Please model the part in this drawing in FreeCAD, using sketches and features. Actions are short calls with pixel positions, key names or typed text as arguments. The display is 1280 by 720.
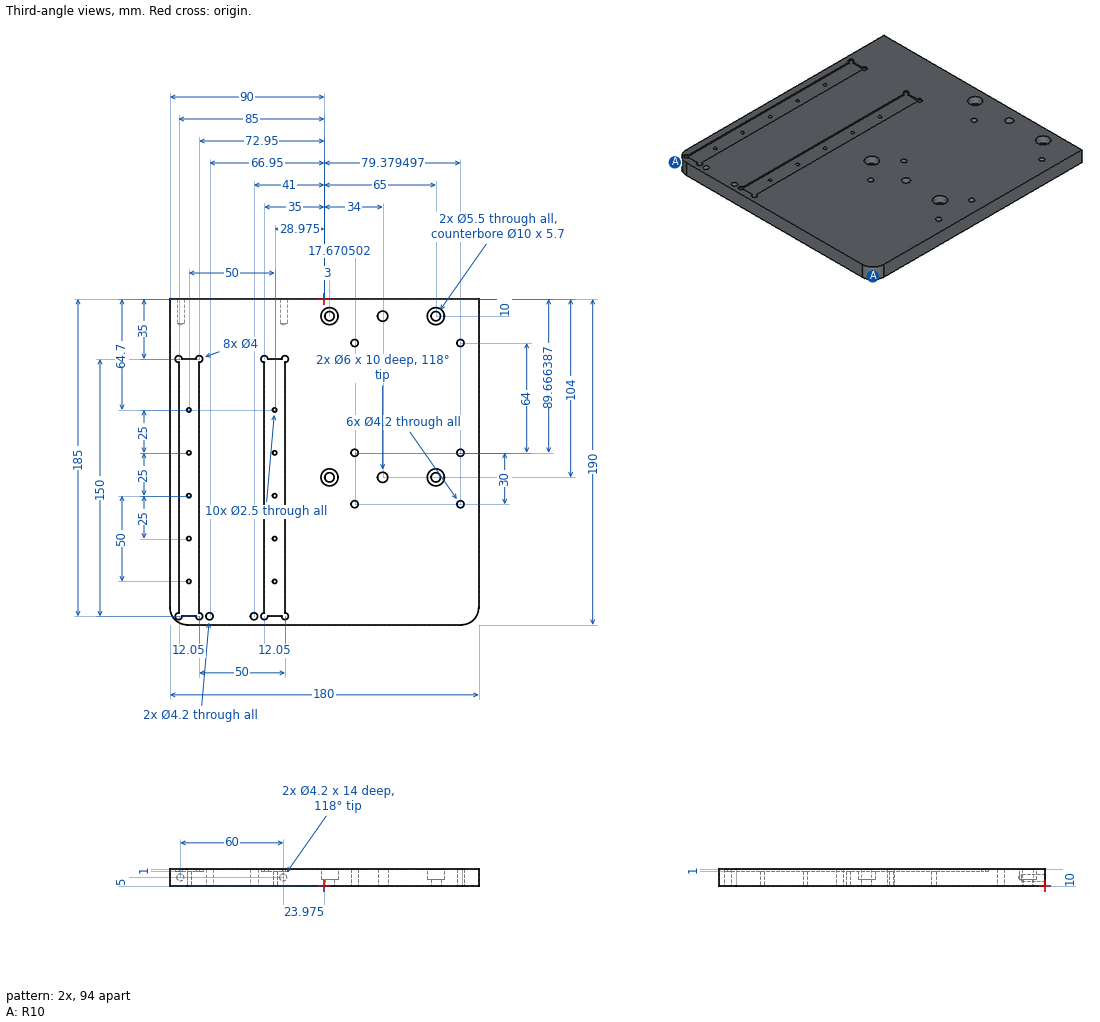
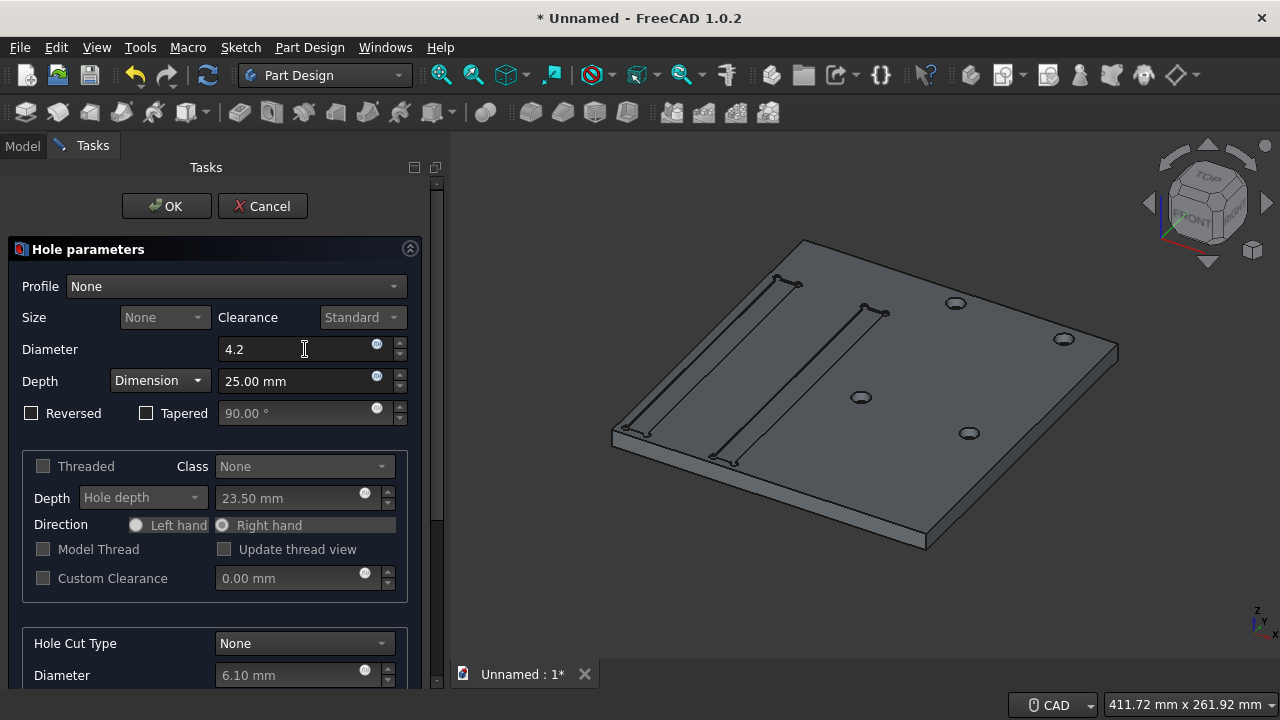
triple_click(305, 381)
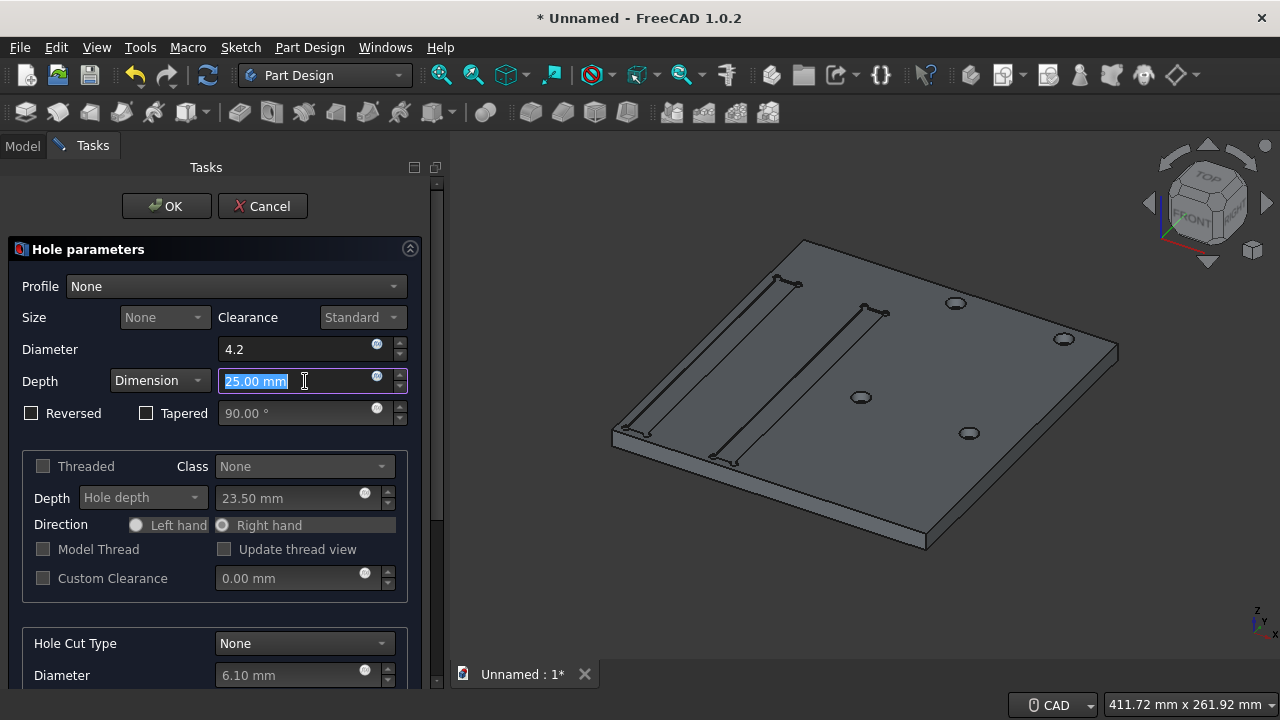
text(14)
key(Tab)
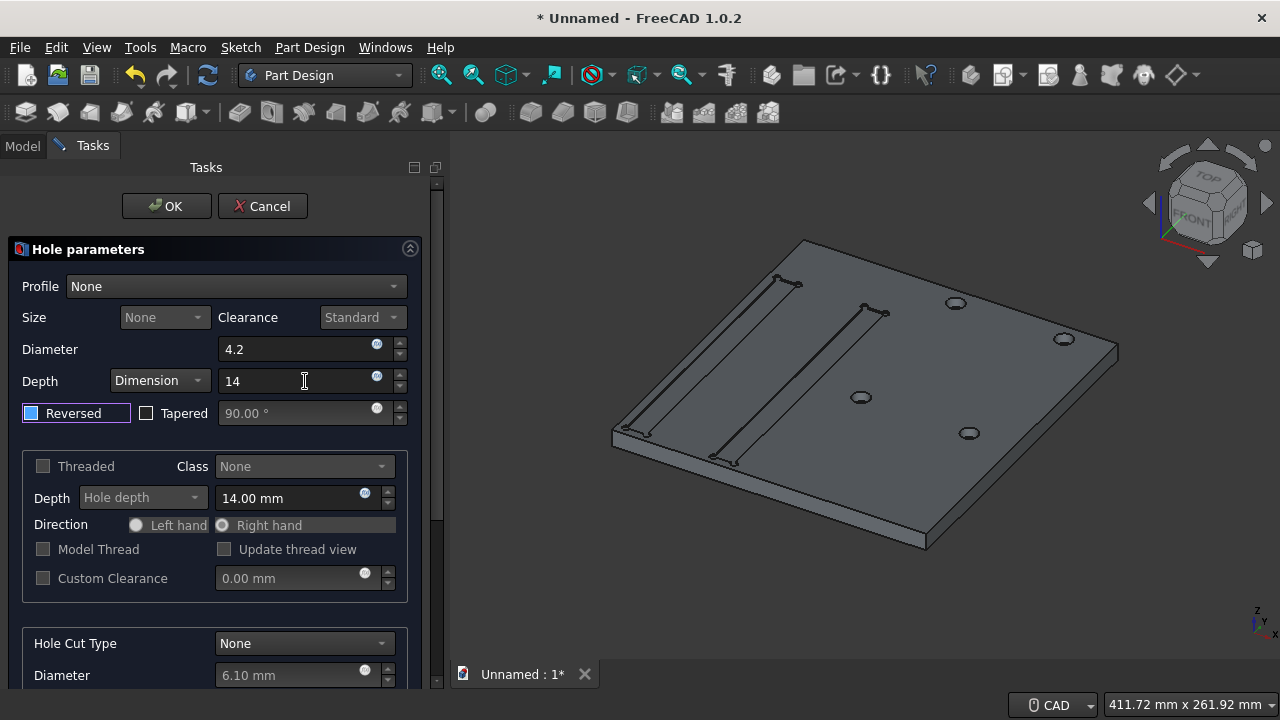
click(30, 413)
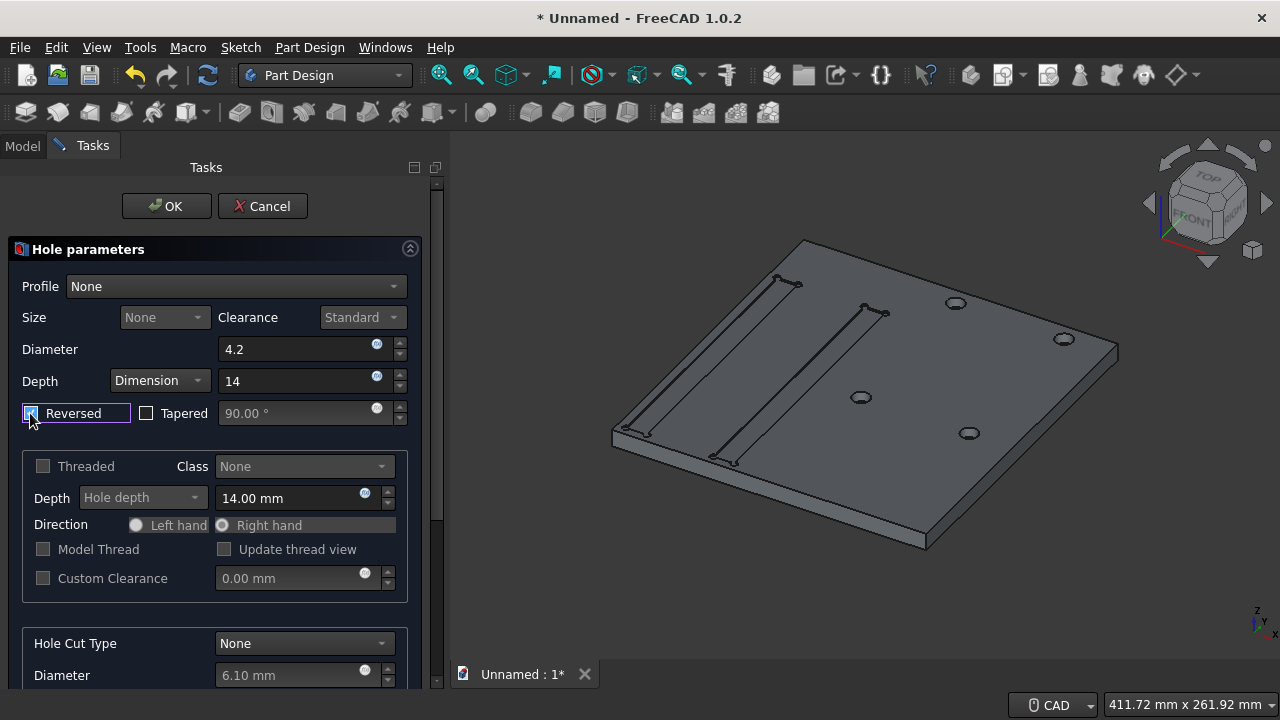
click(167, 206)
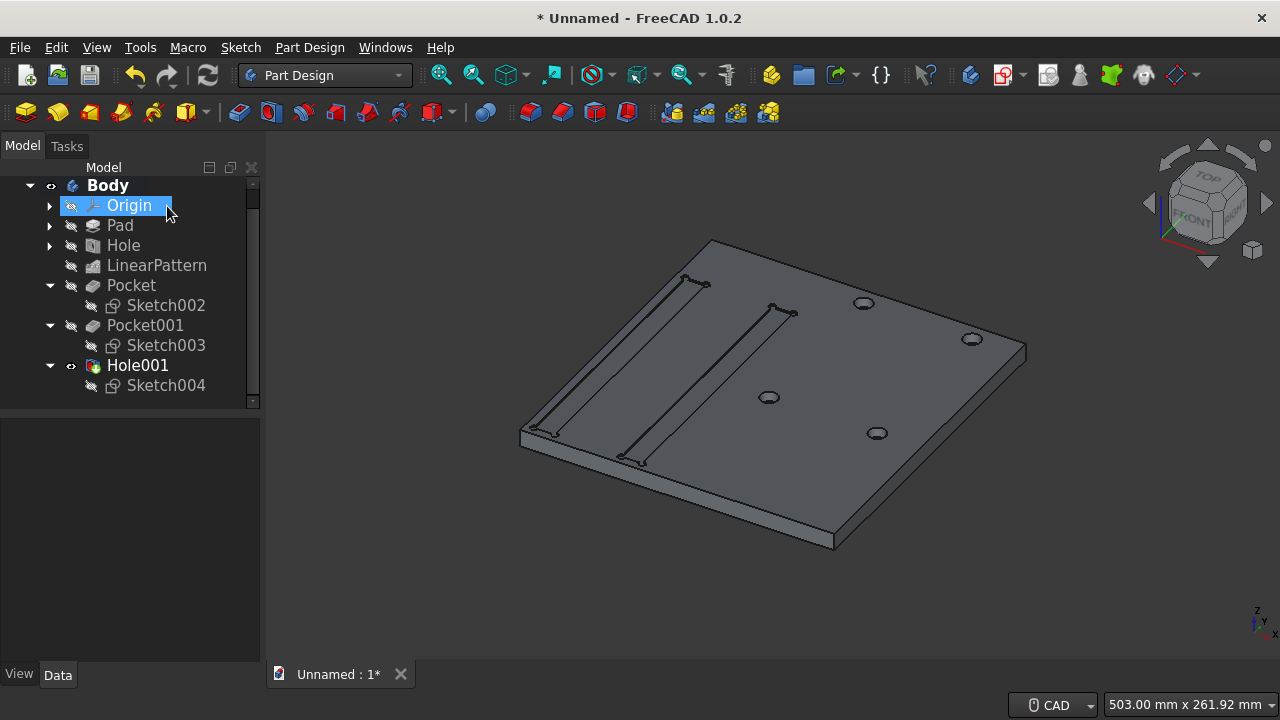
click(834, 541)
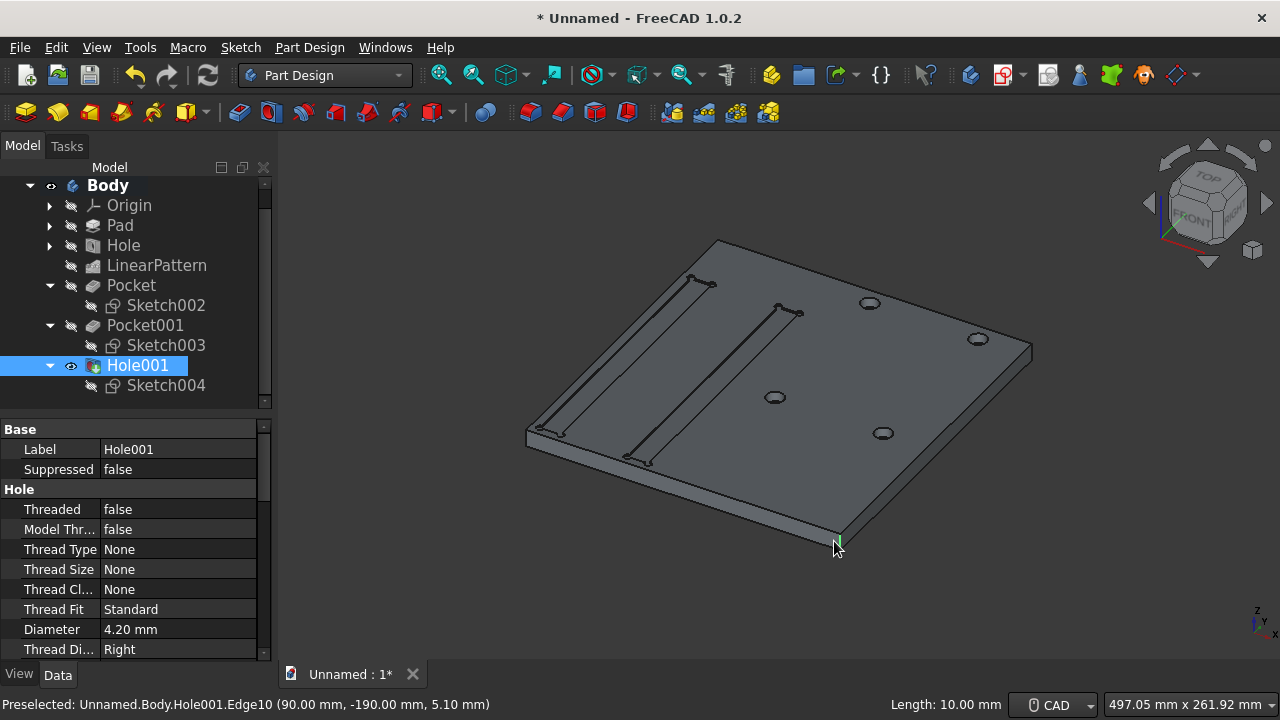
scroll(526, 437, up, 4)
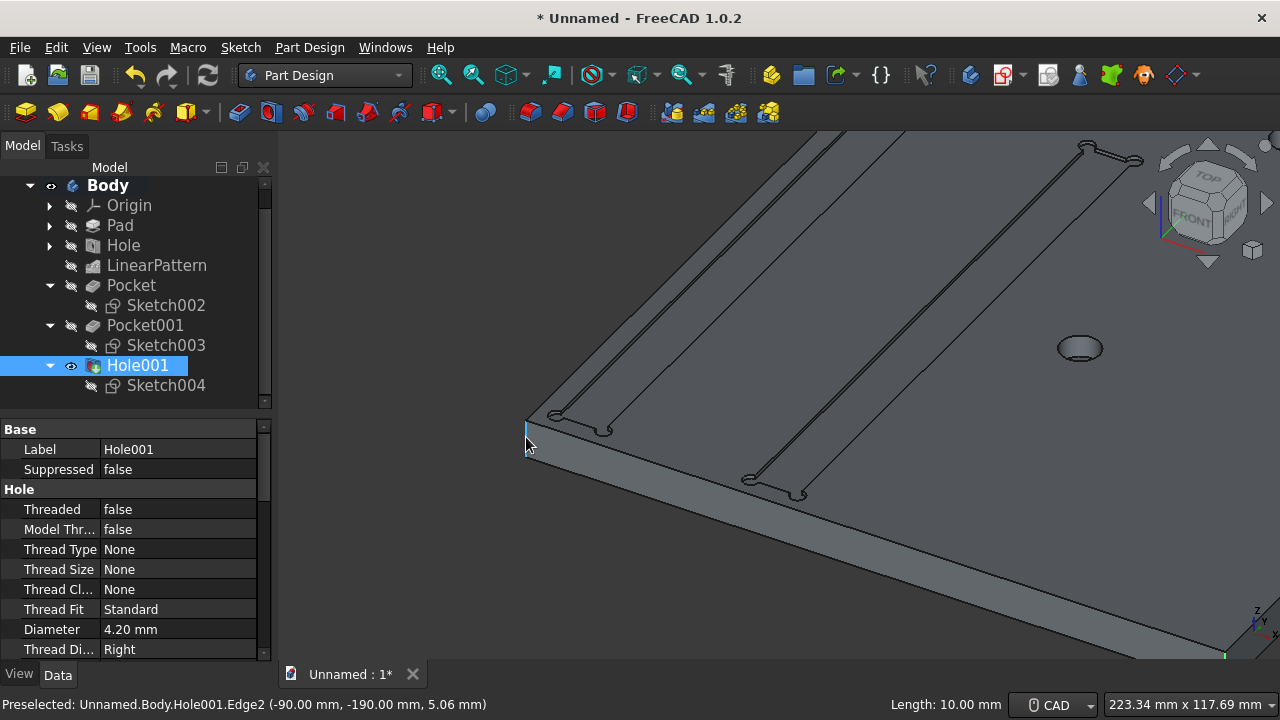
key(v)
key(f)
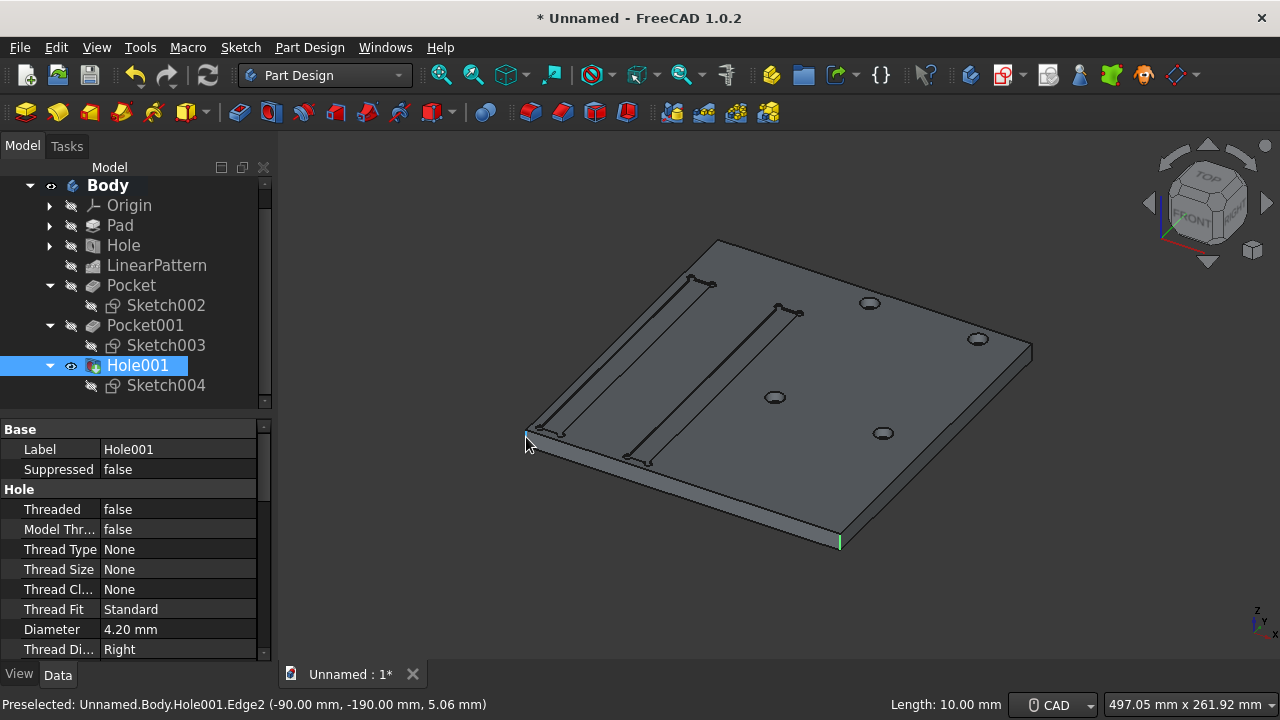
key(0)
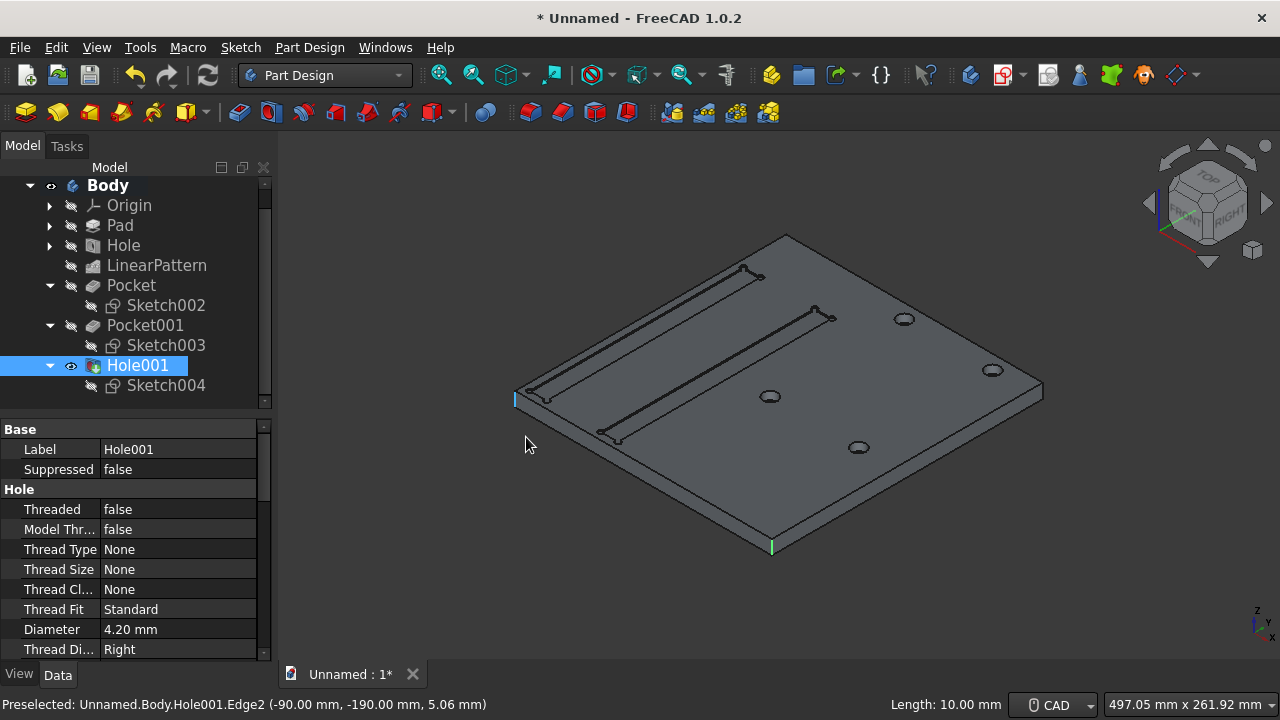
scroll(515, 398, up, 4)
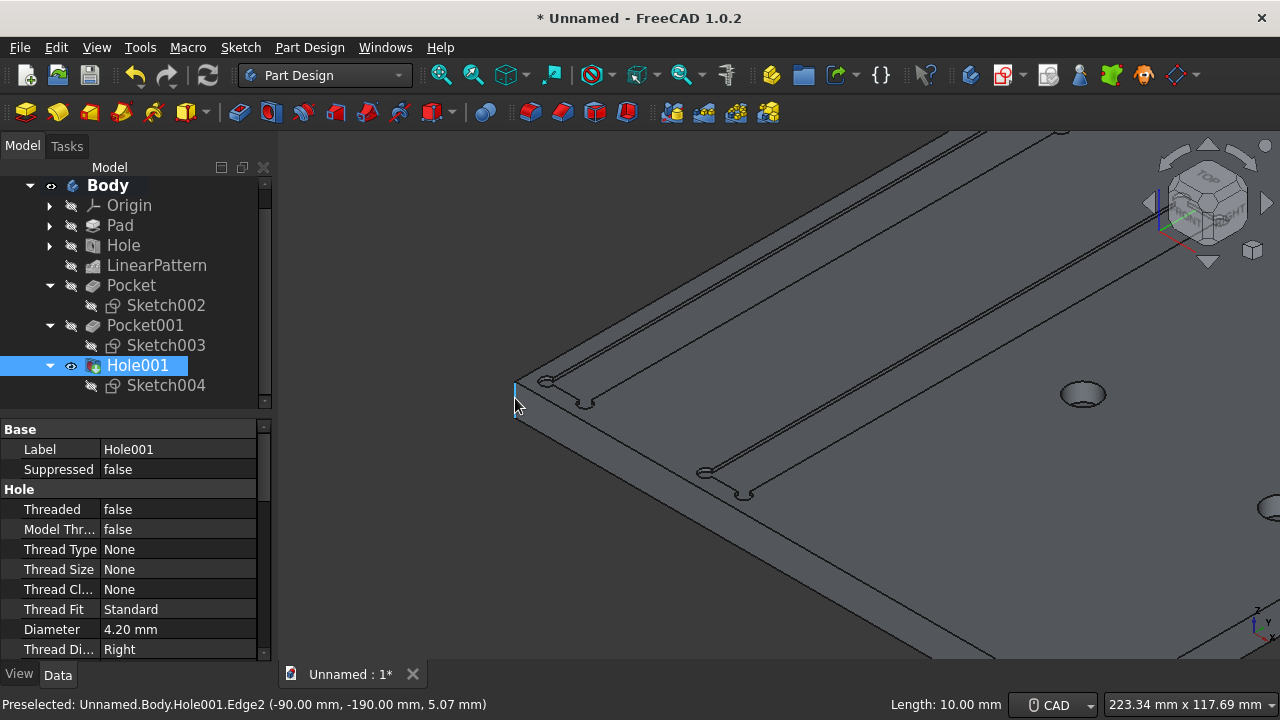
key(v)
key(f)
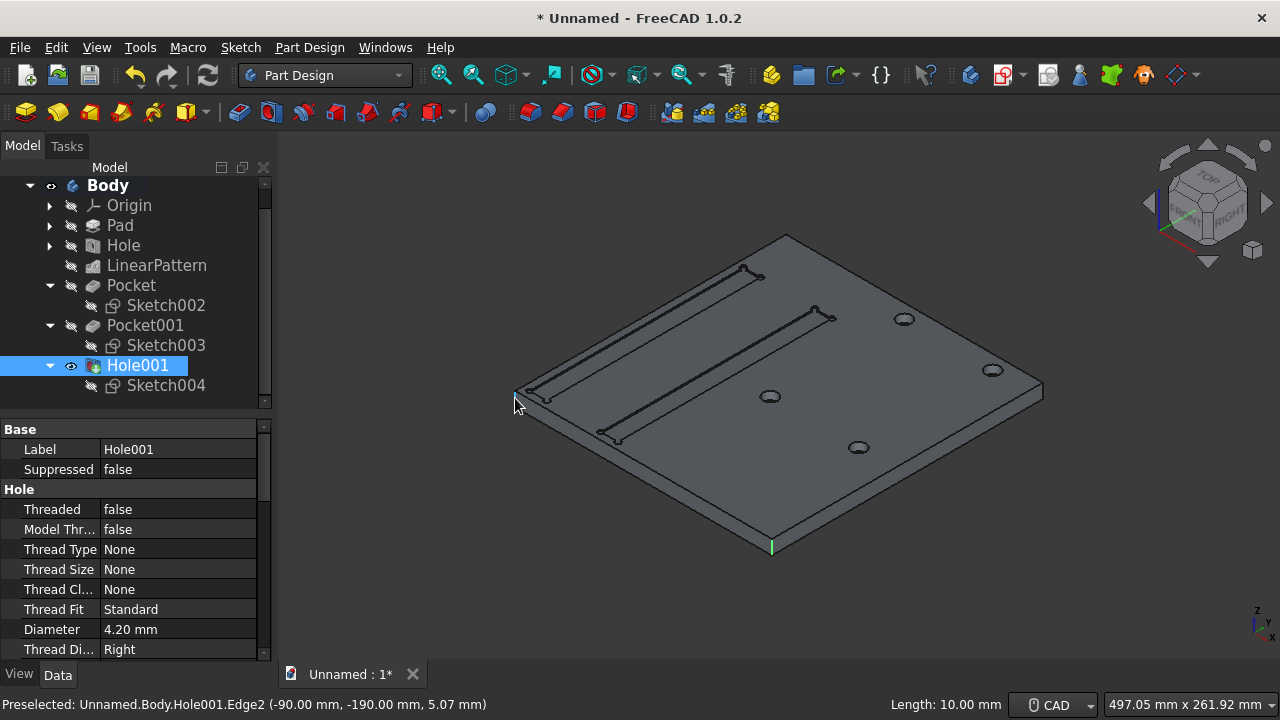
key(2)